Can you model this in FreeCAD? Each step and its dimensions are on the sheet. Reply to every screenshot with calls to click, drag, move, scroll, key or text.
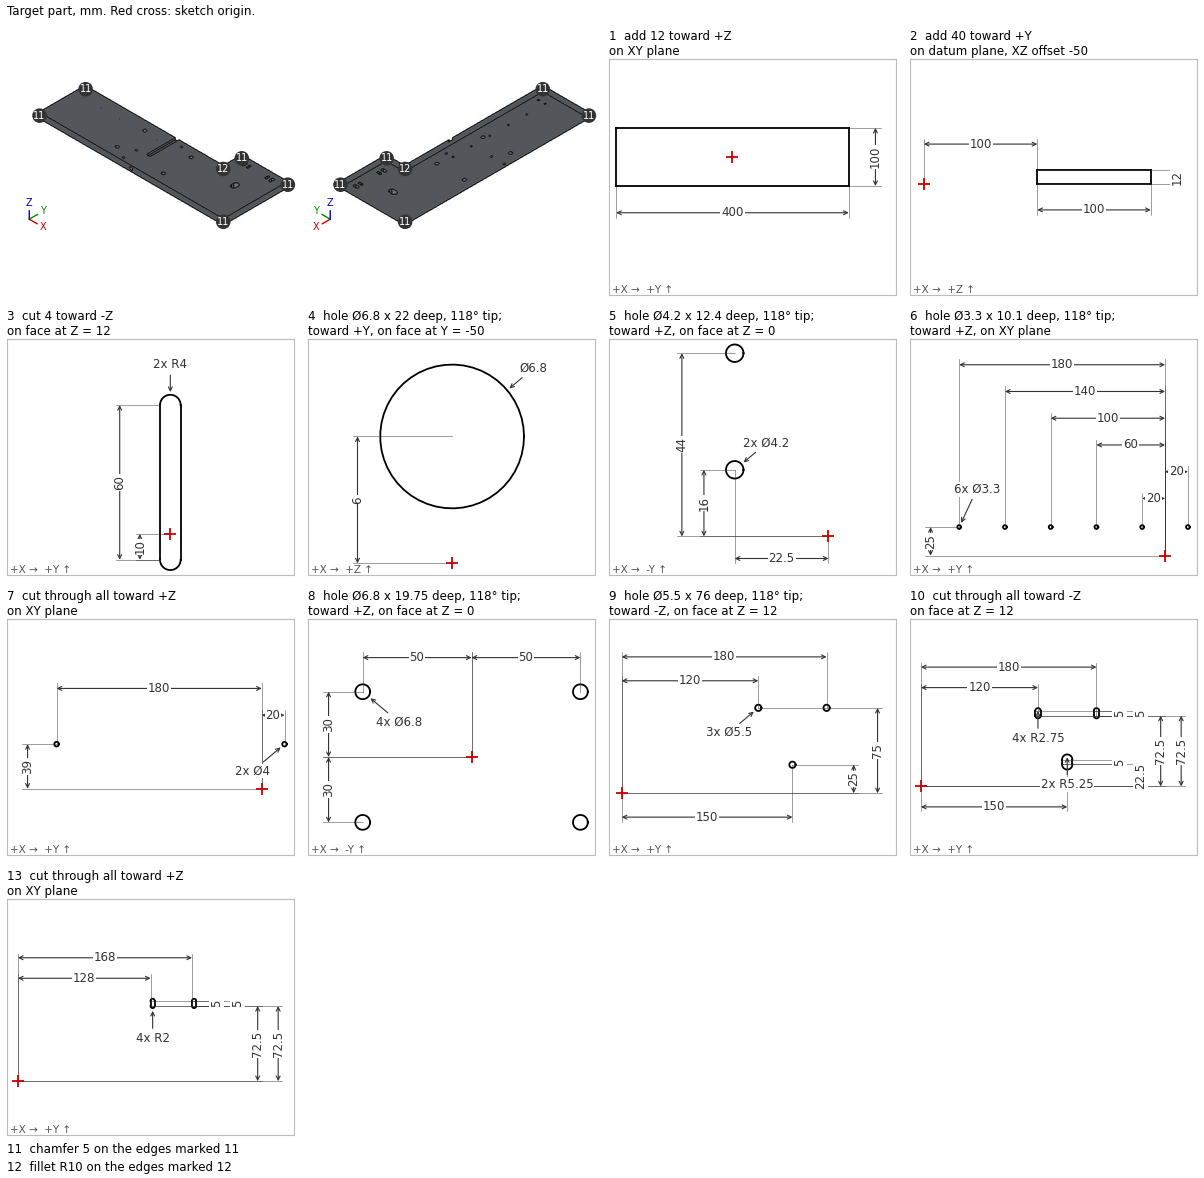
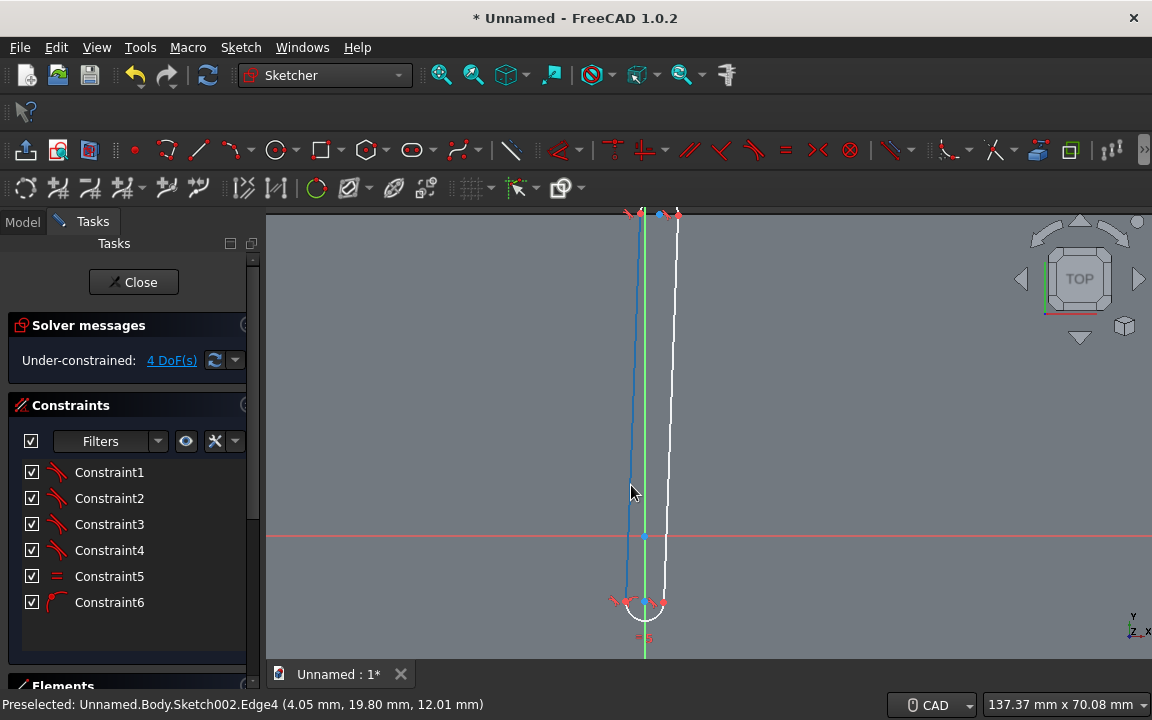
click(630, 485)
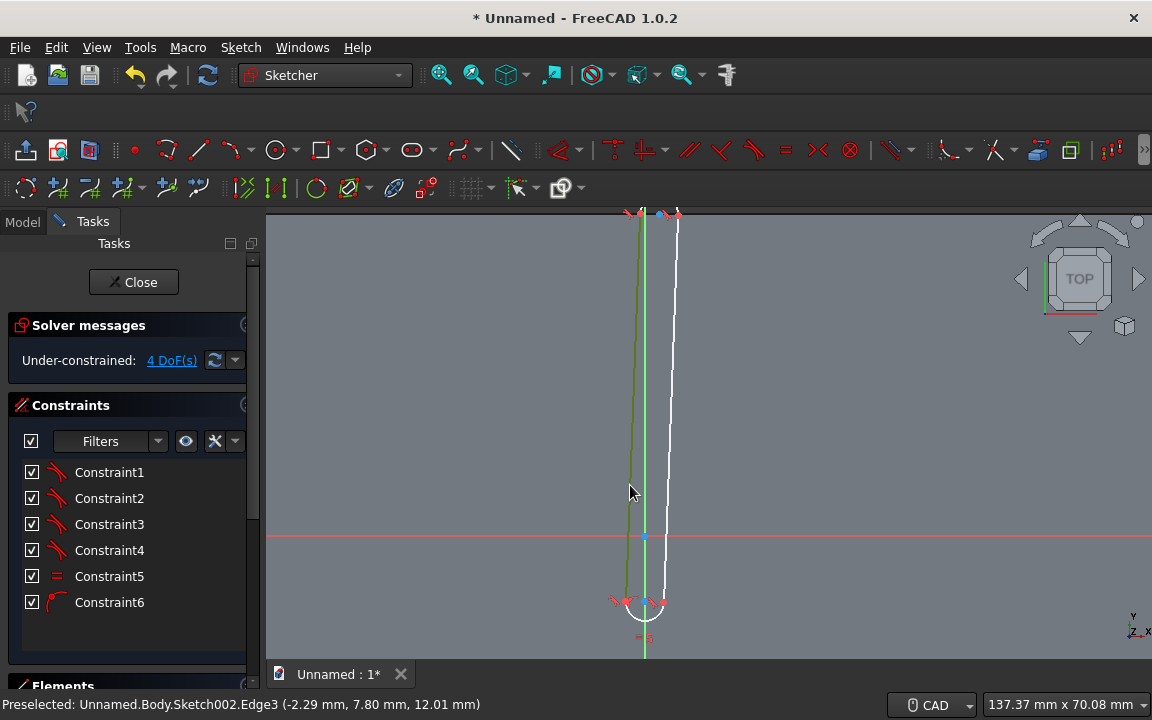
key(v)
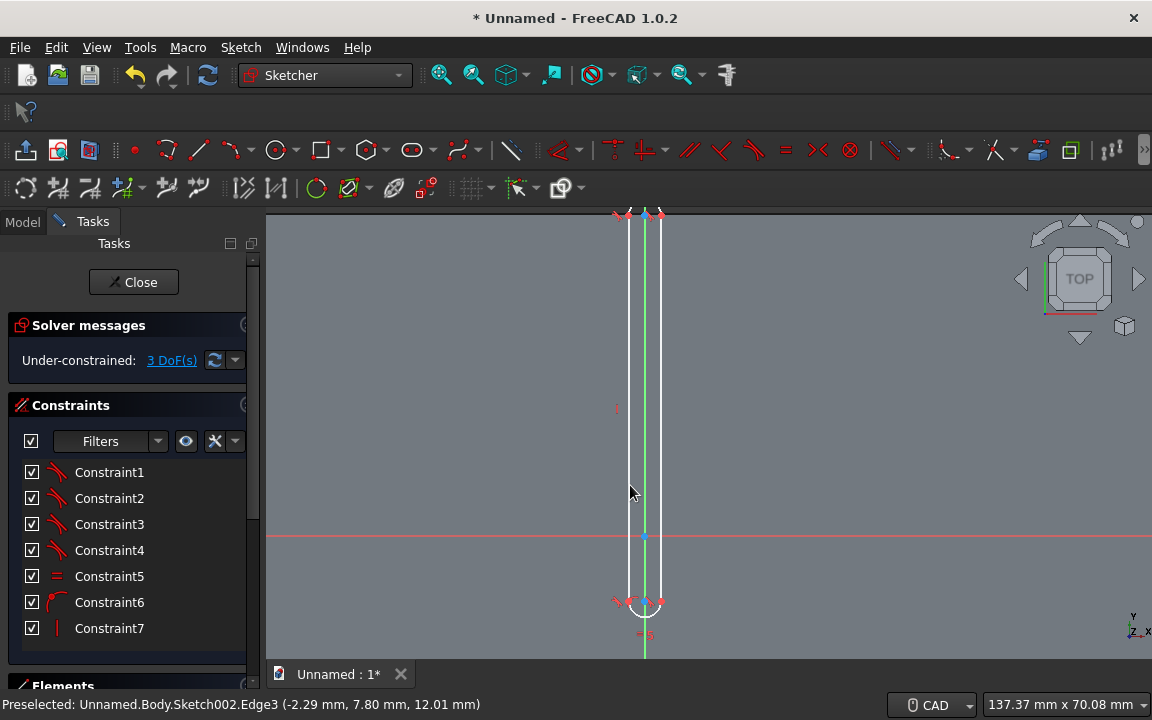
click(558, 150)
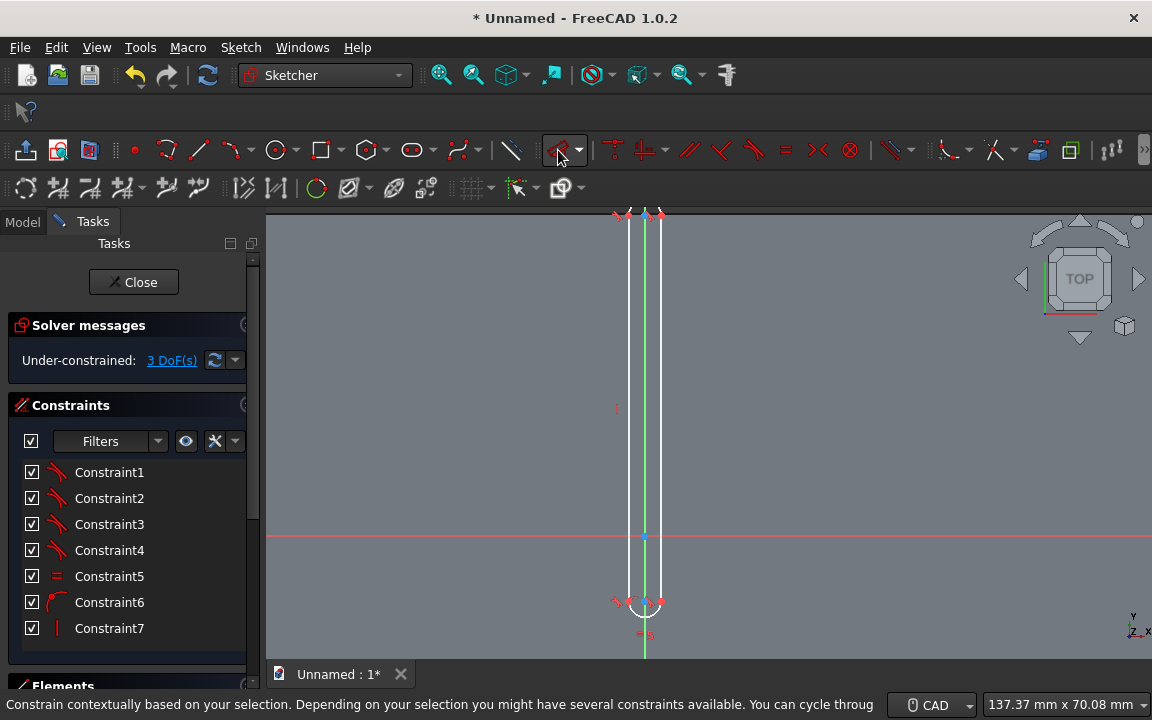
scroll(636, 614, up, 3)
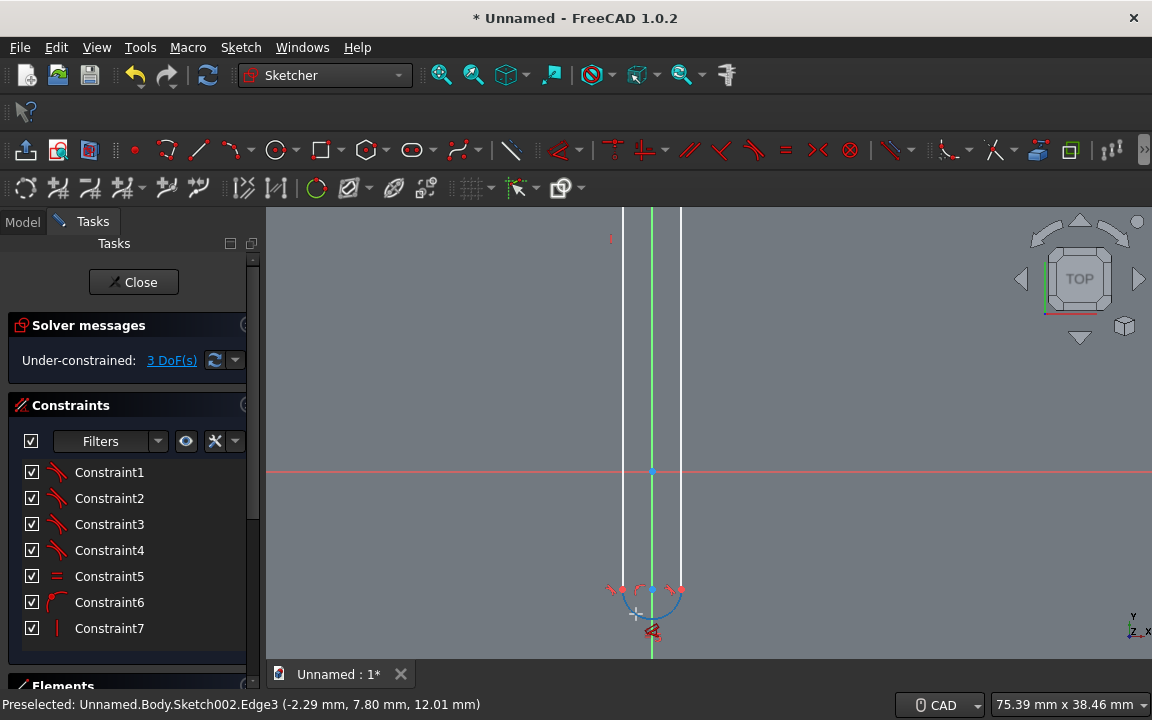
click(635, 614)
click(597, 617)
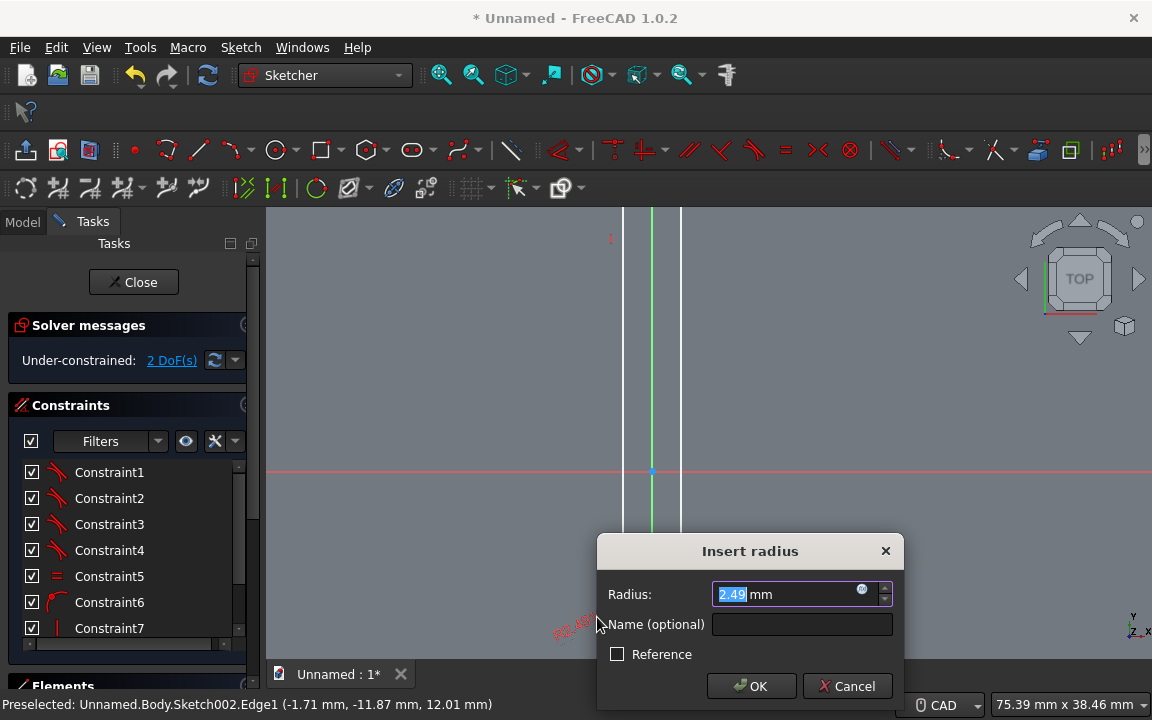
text(4)
key(Return)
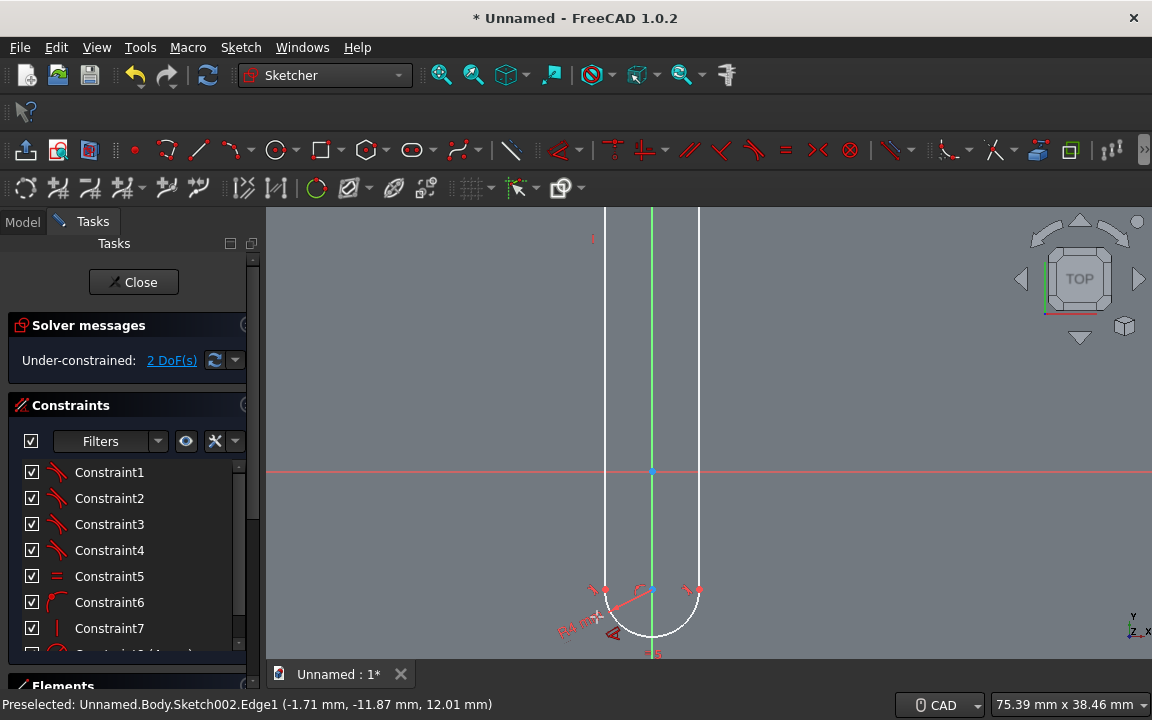
click(605, 379)
click(571, 412)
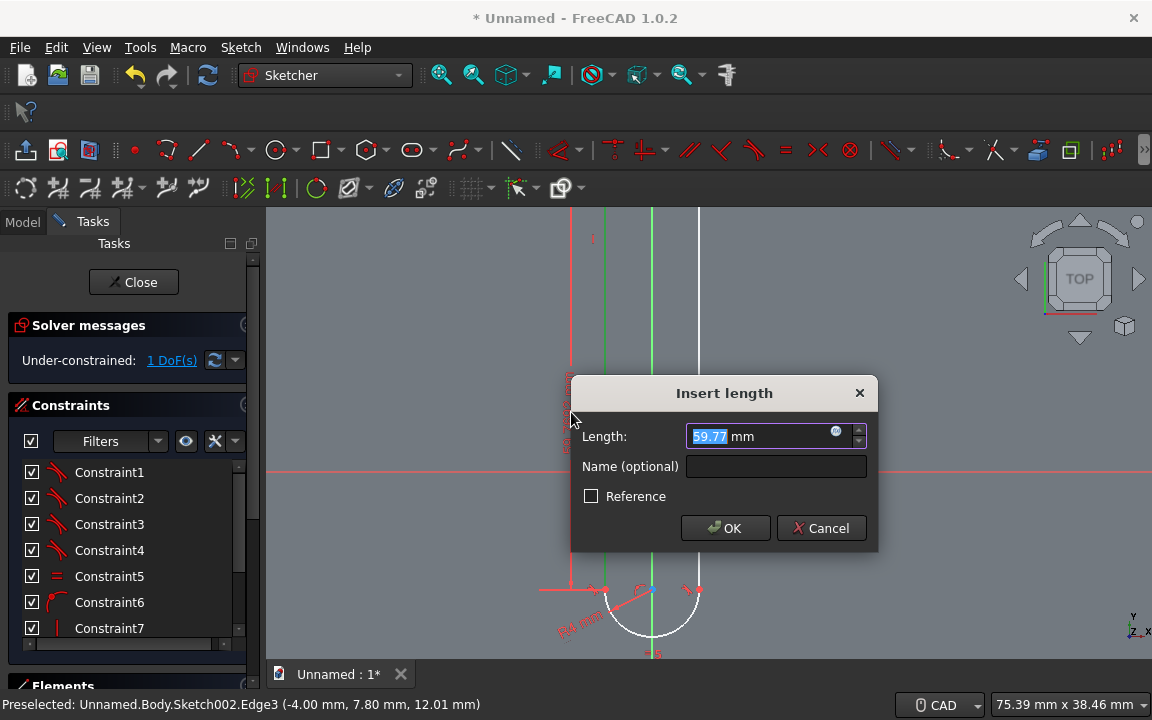
text(60)
key(Return)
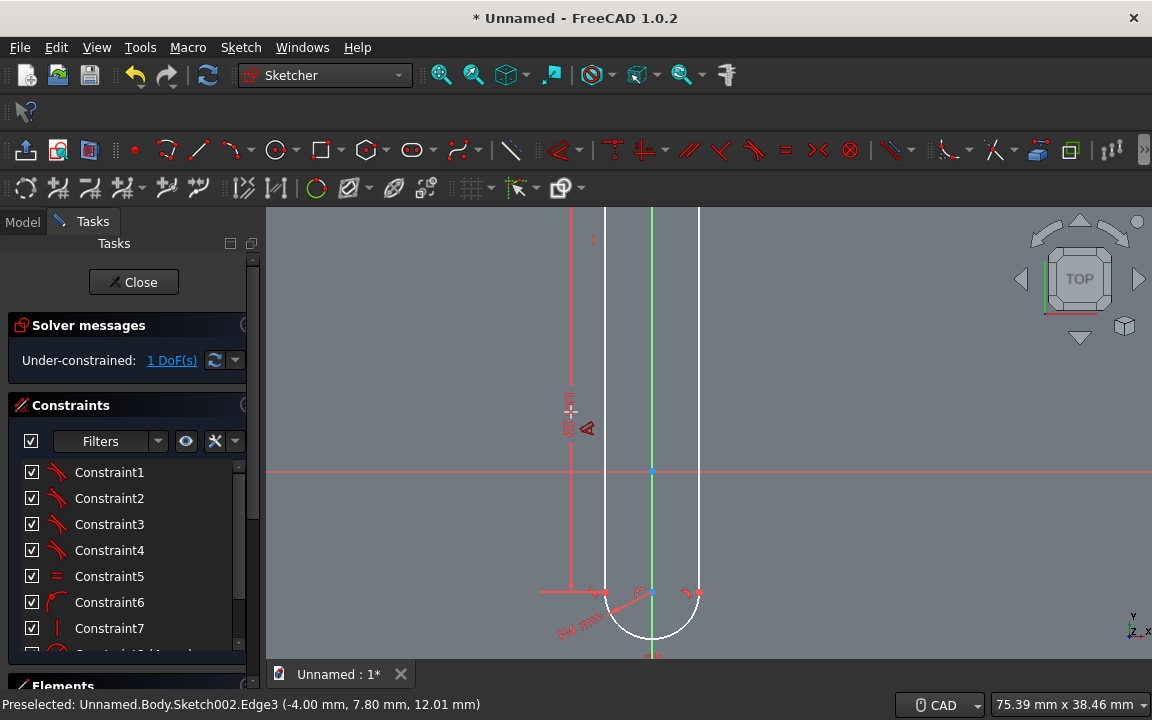
click(605, 592)
click(571, 532)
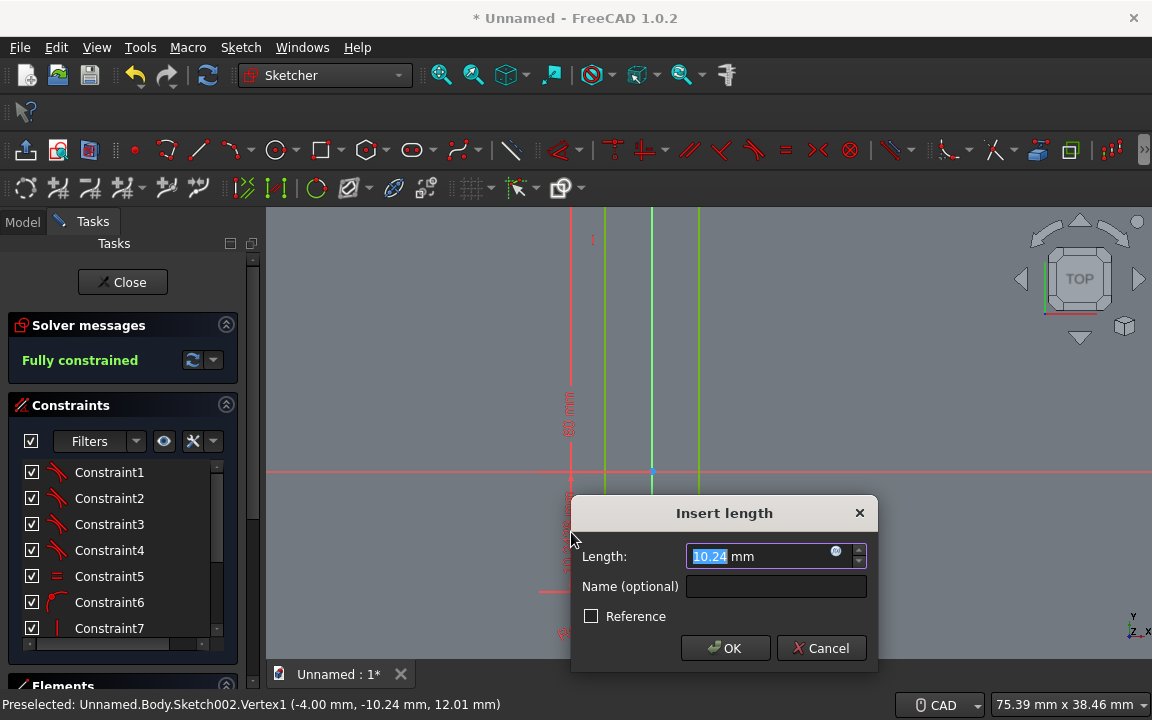
text(10)
key(Return)
key(Escape)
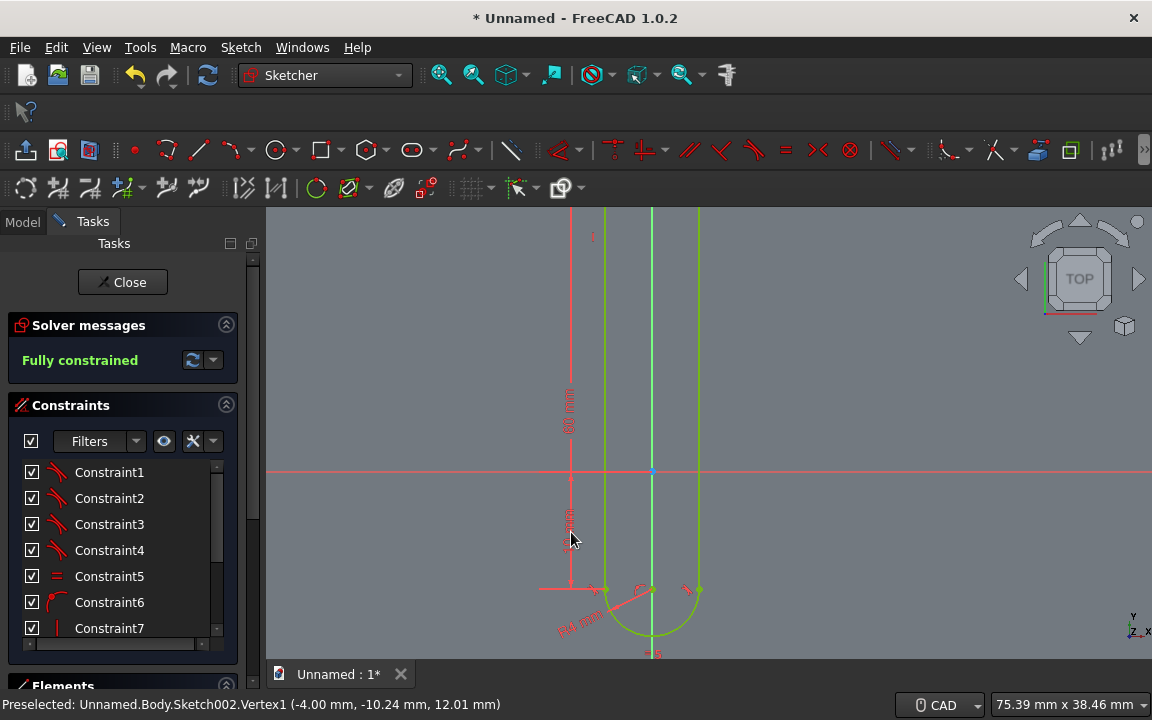
click(123, 282)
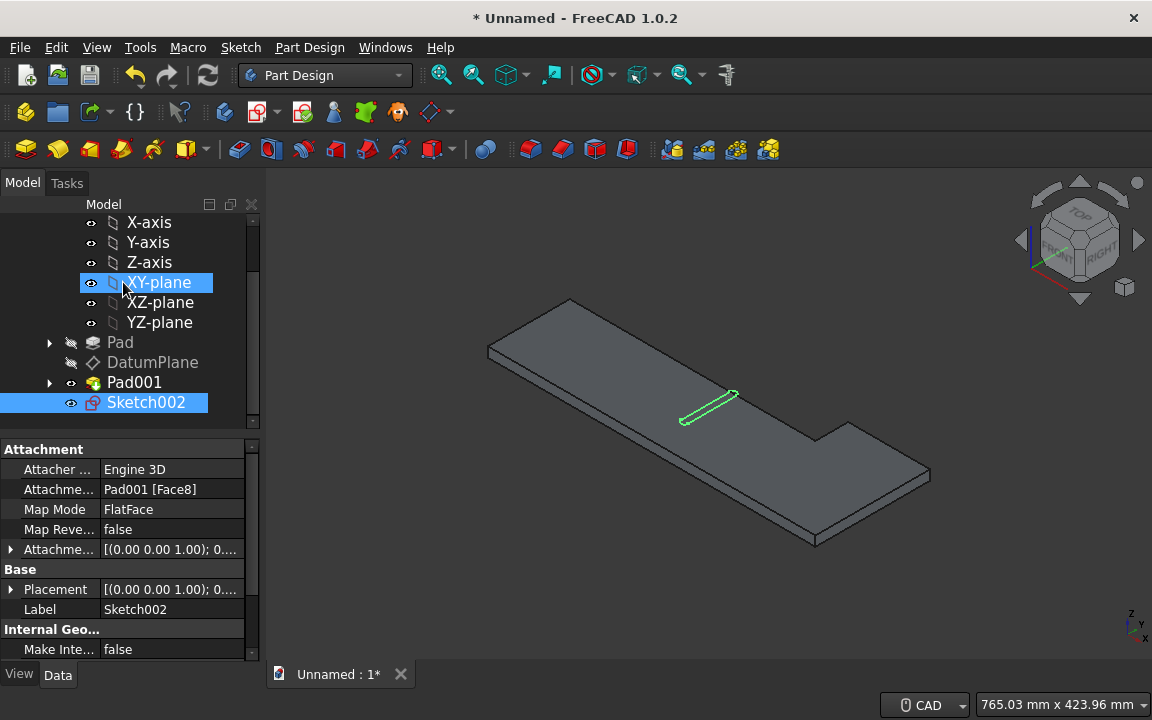
click(240, 150)